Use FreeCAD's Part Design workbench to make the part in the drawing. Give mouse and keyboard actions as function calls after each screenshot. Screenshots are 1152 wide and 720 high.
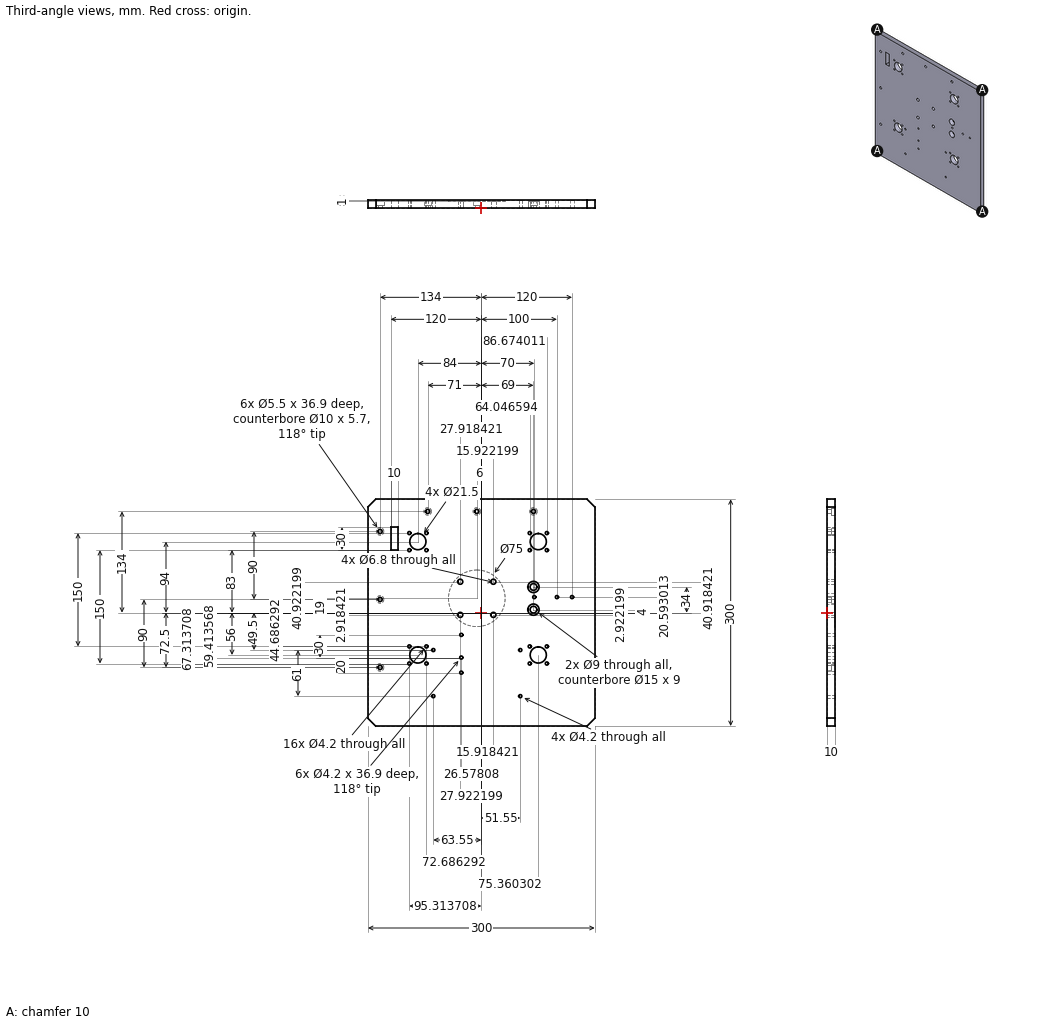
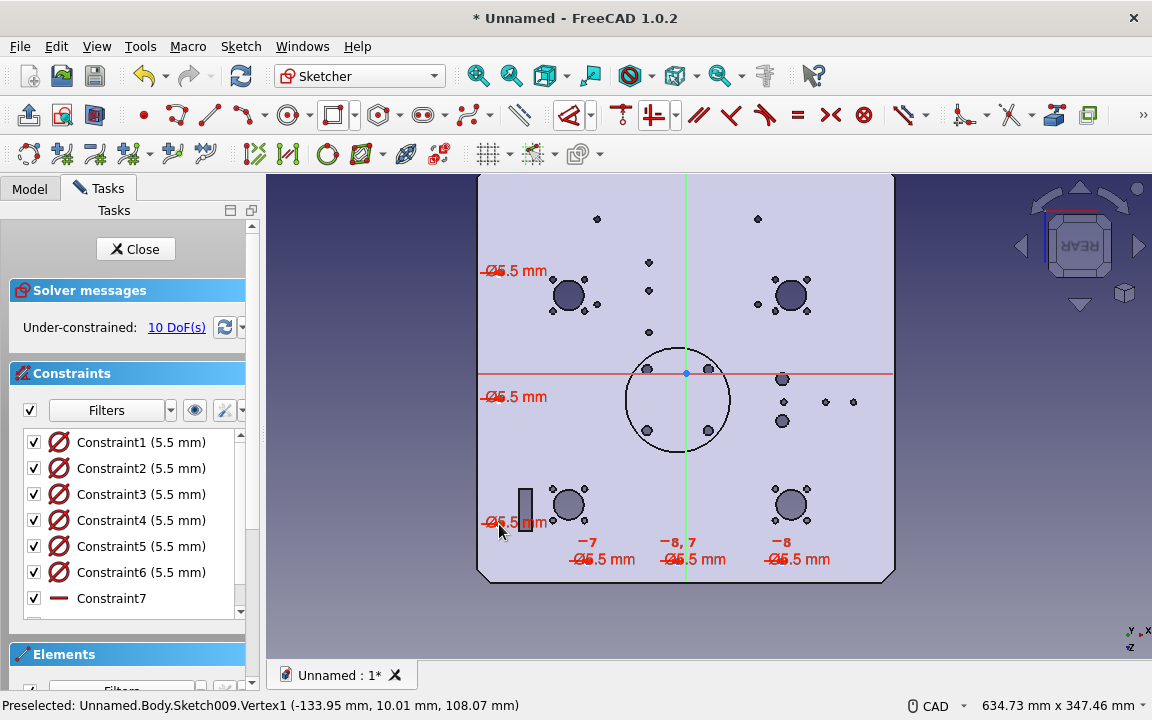
click(499, 273)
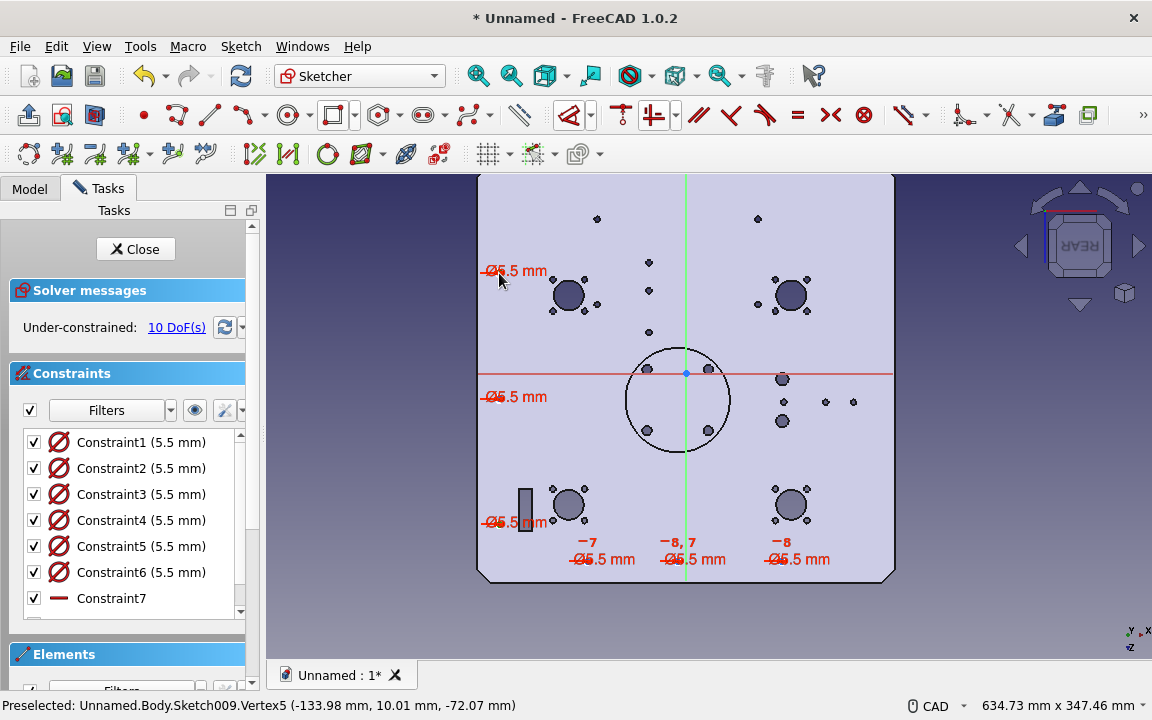
click(676, 116)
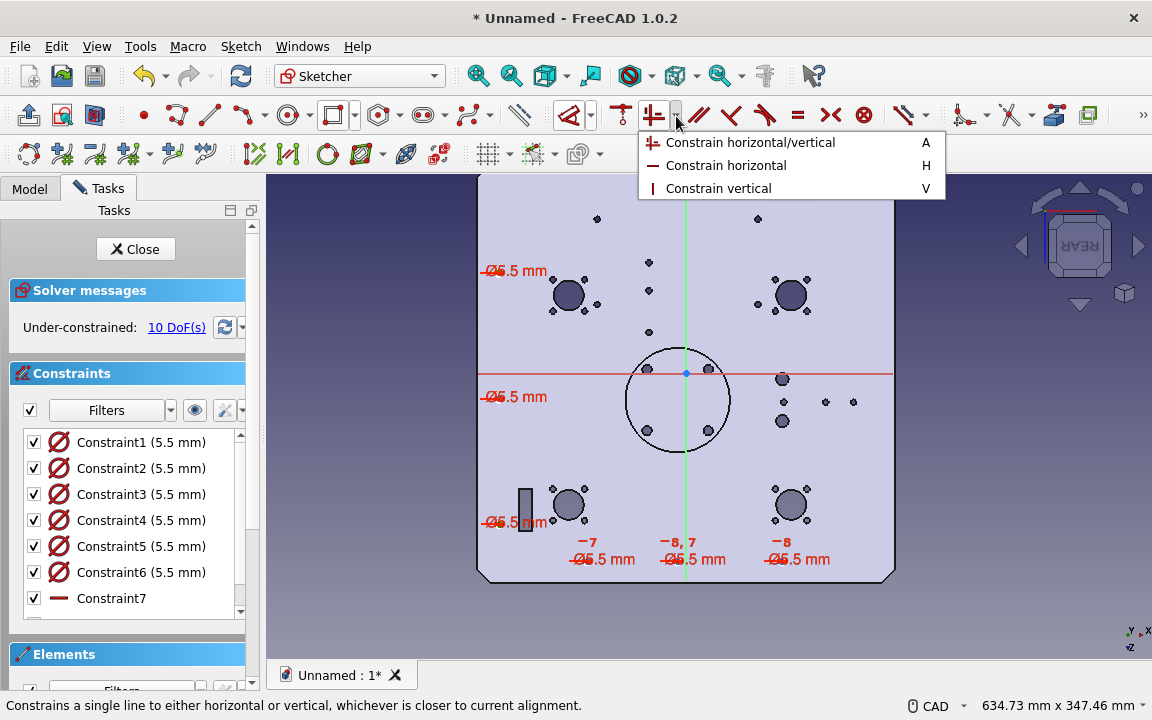
click(792, 188)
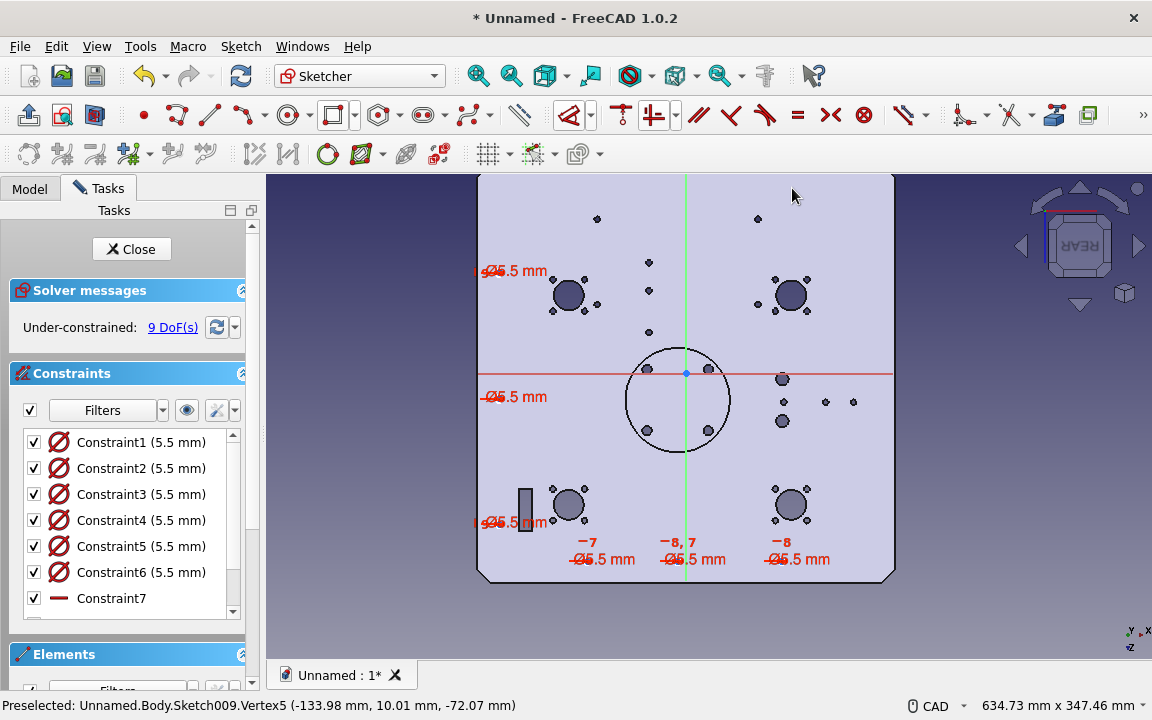
click(499, 524)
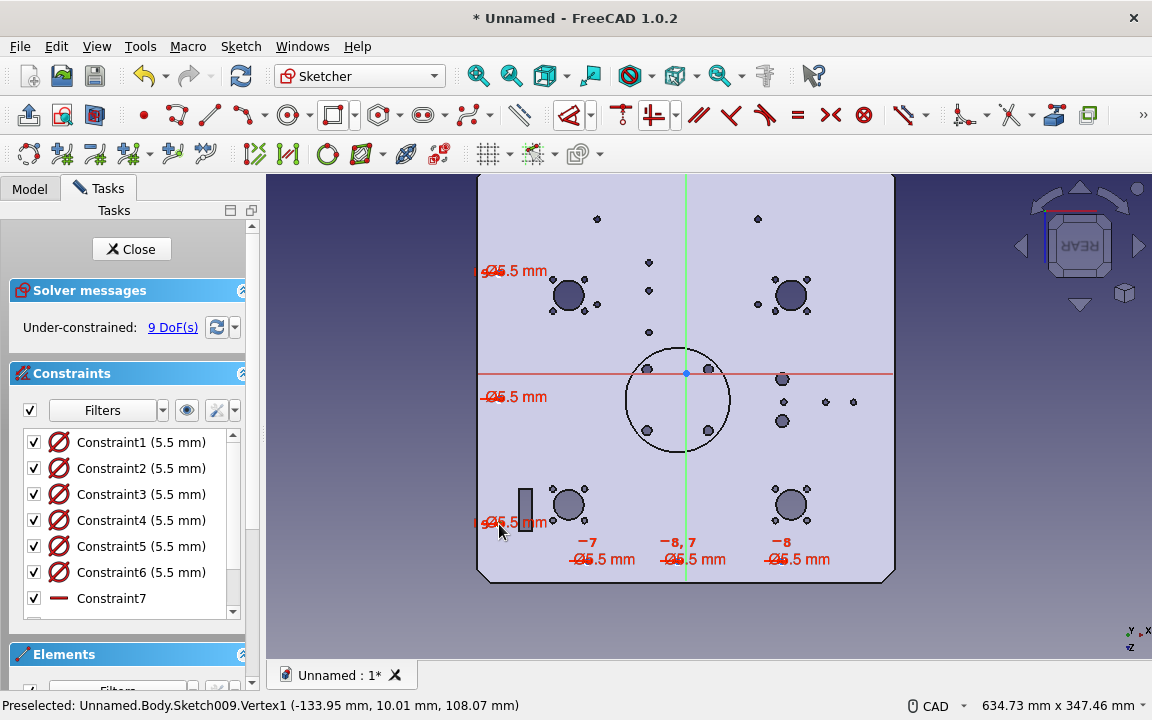
click(499, 399)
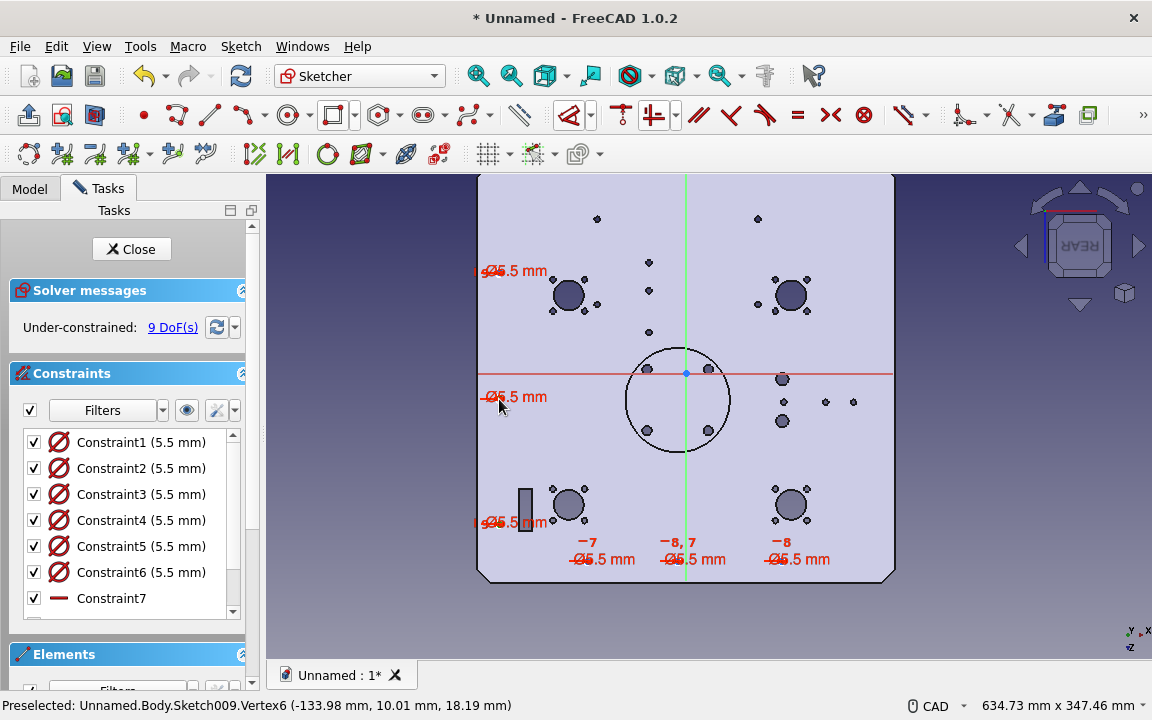
key(v)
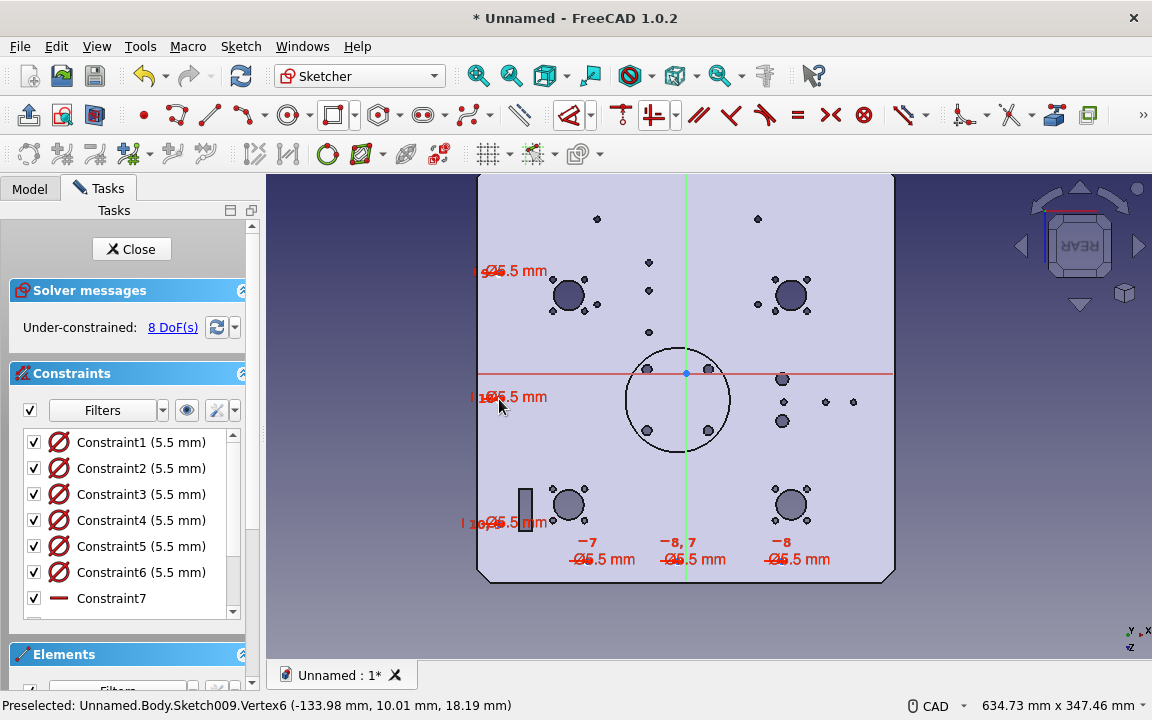
scroll(678, 561, up, 8)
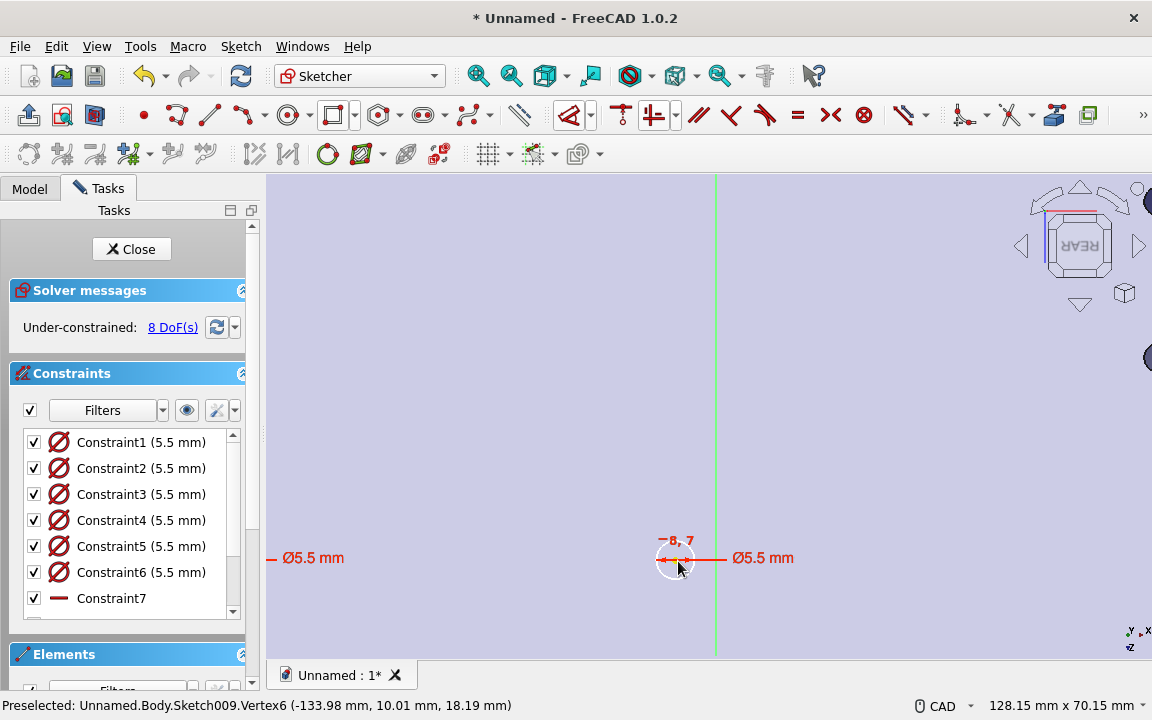
click(675, 560)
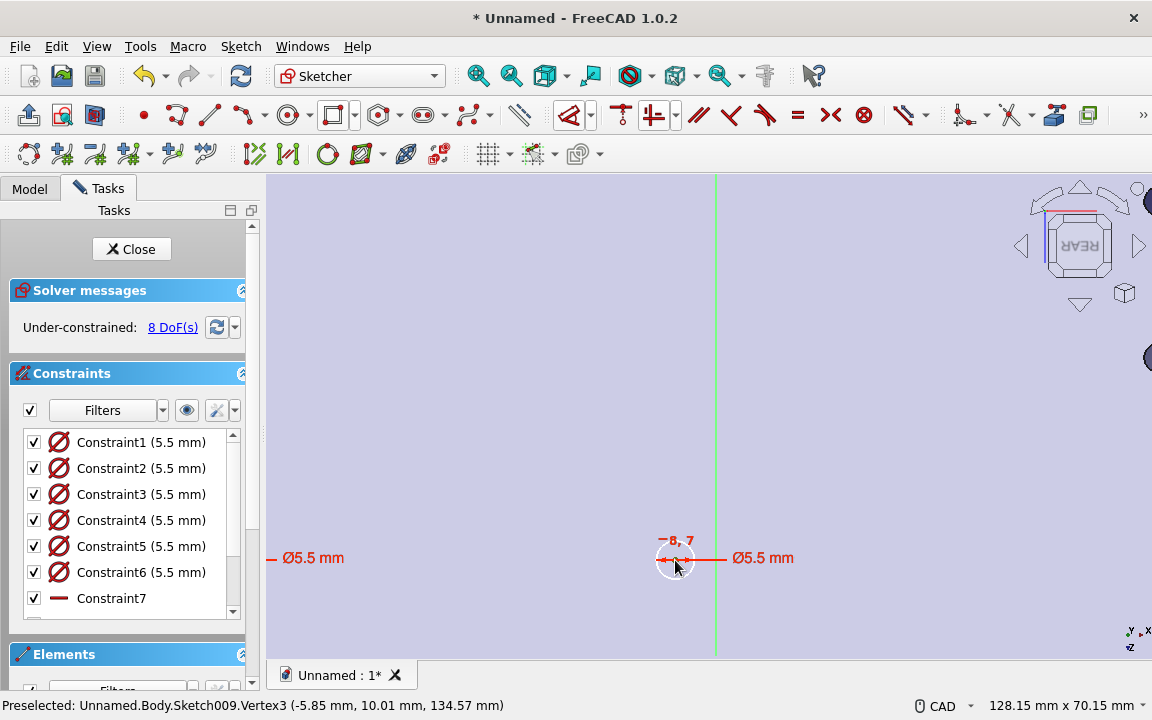
click(590, 116)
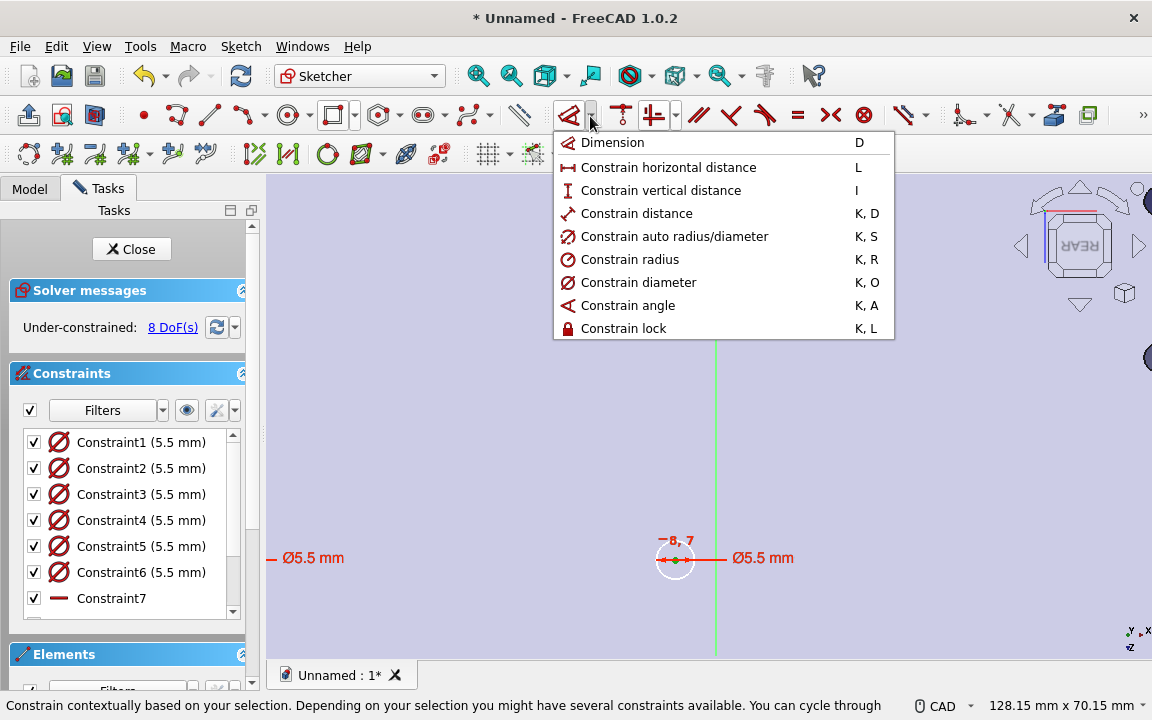
click(724, 168)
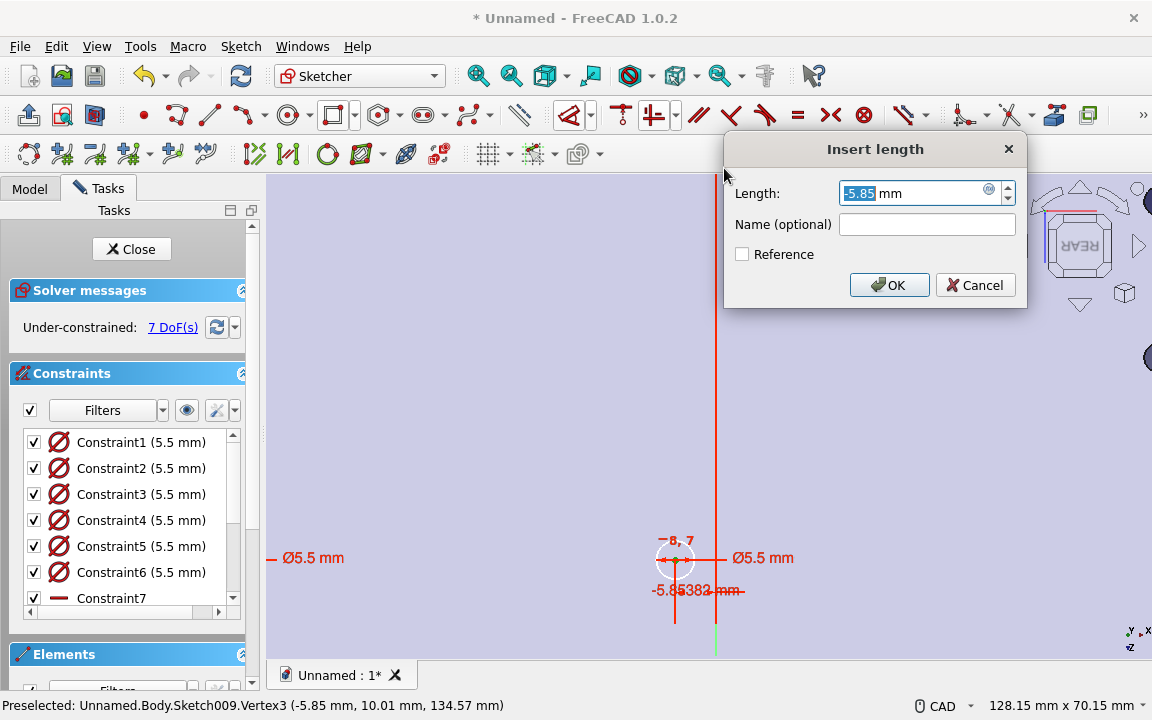
text(-6)
key(Return)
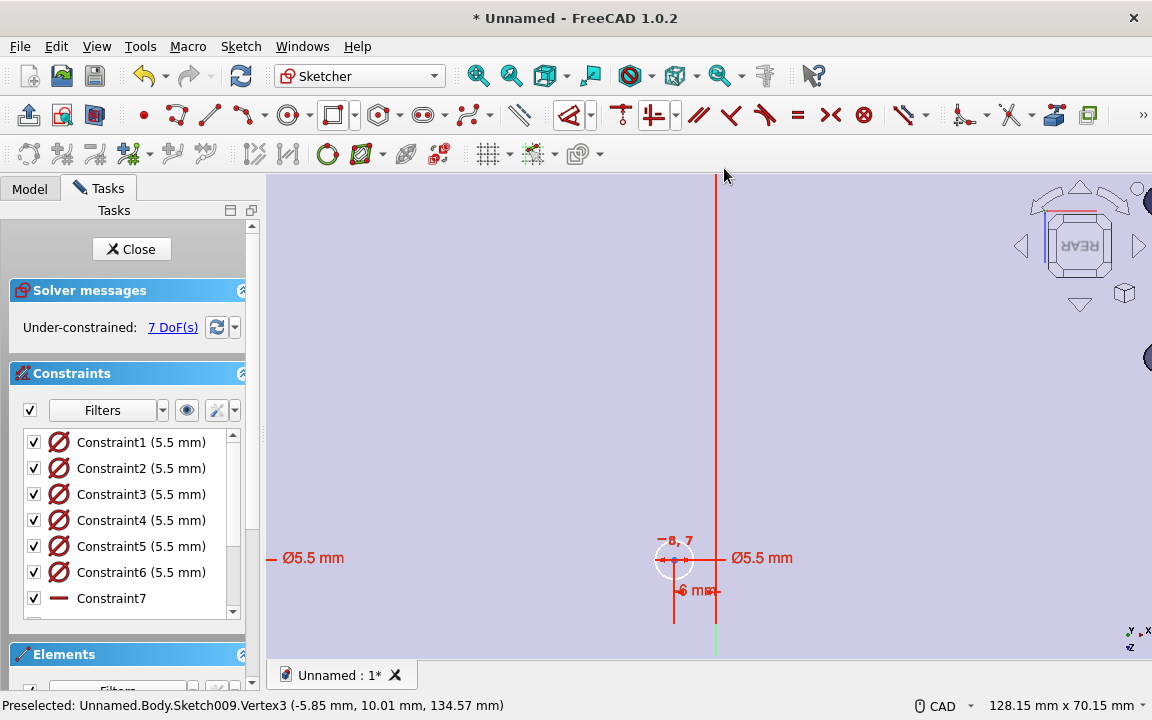
scroll(678, 562, down, 8)